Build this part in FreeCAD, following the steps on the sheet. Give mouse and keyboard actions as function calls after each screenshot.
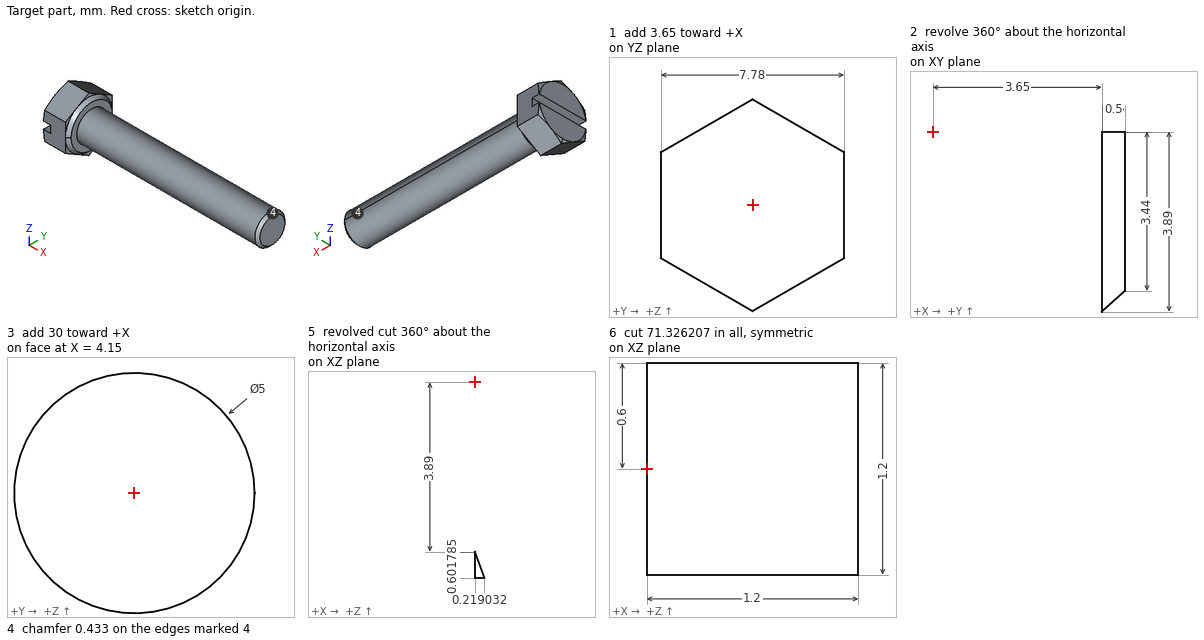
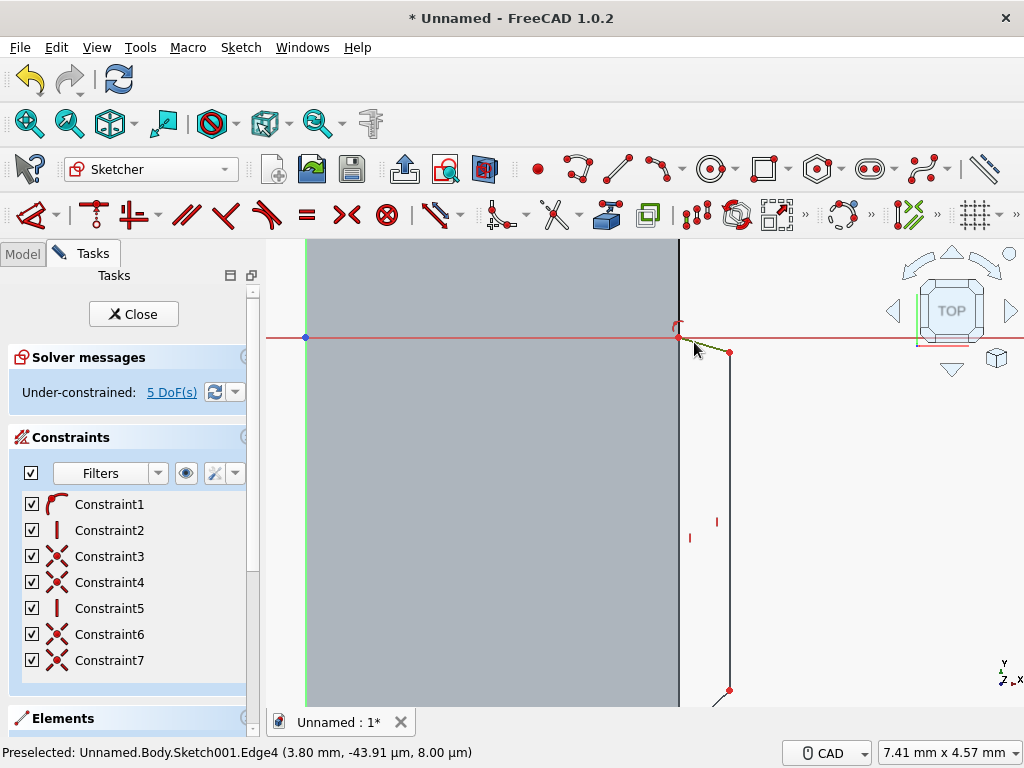
key(h)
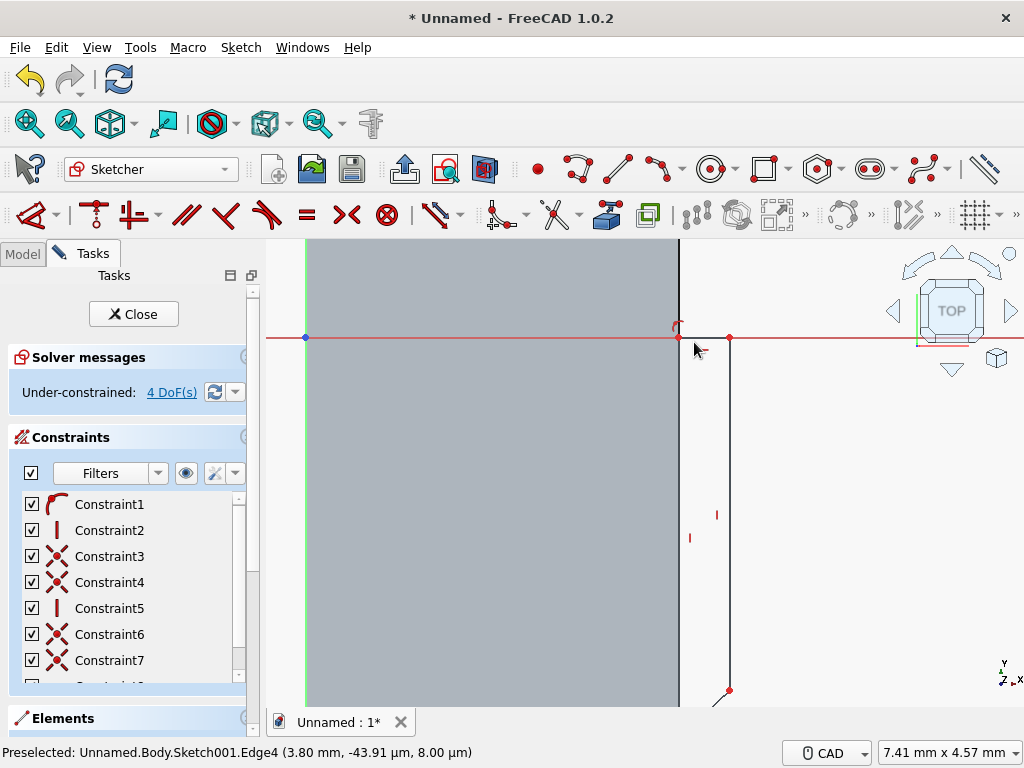
click(714, 338)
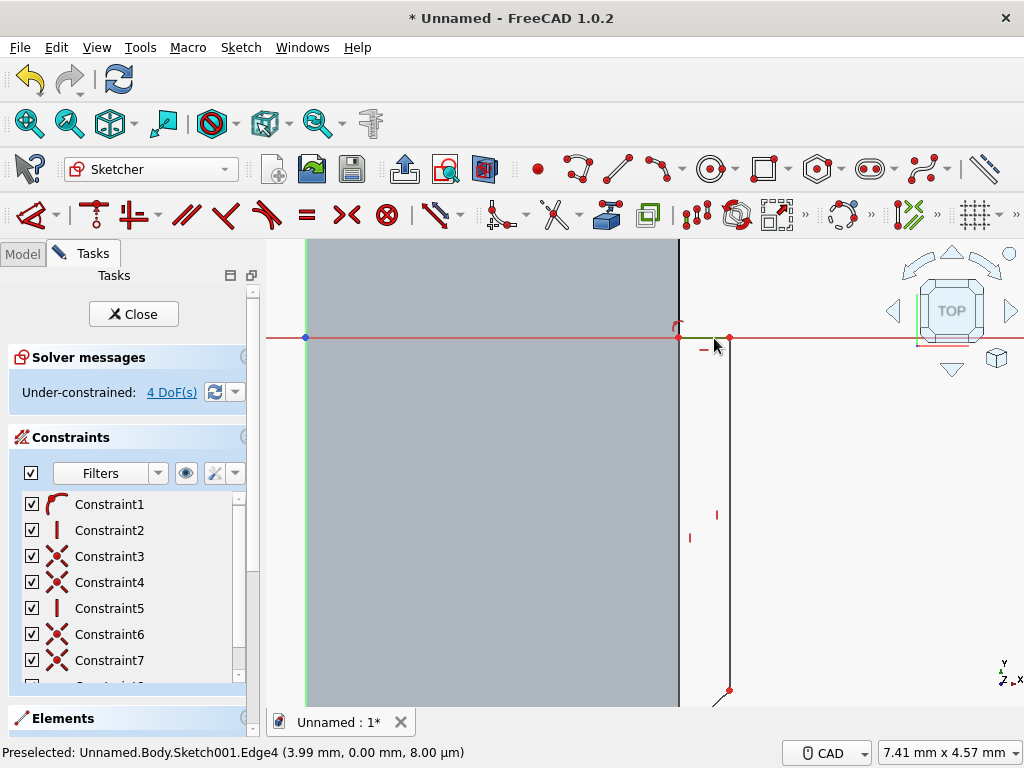
key(l)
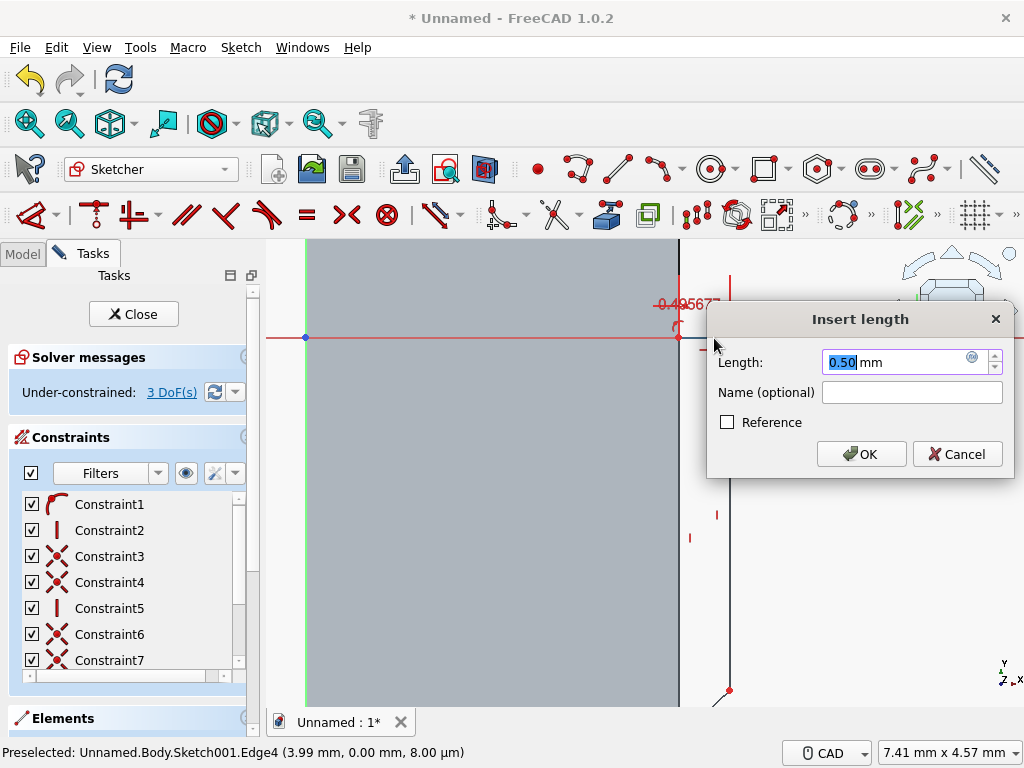
text(0.5)
key(Return)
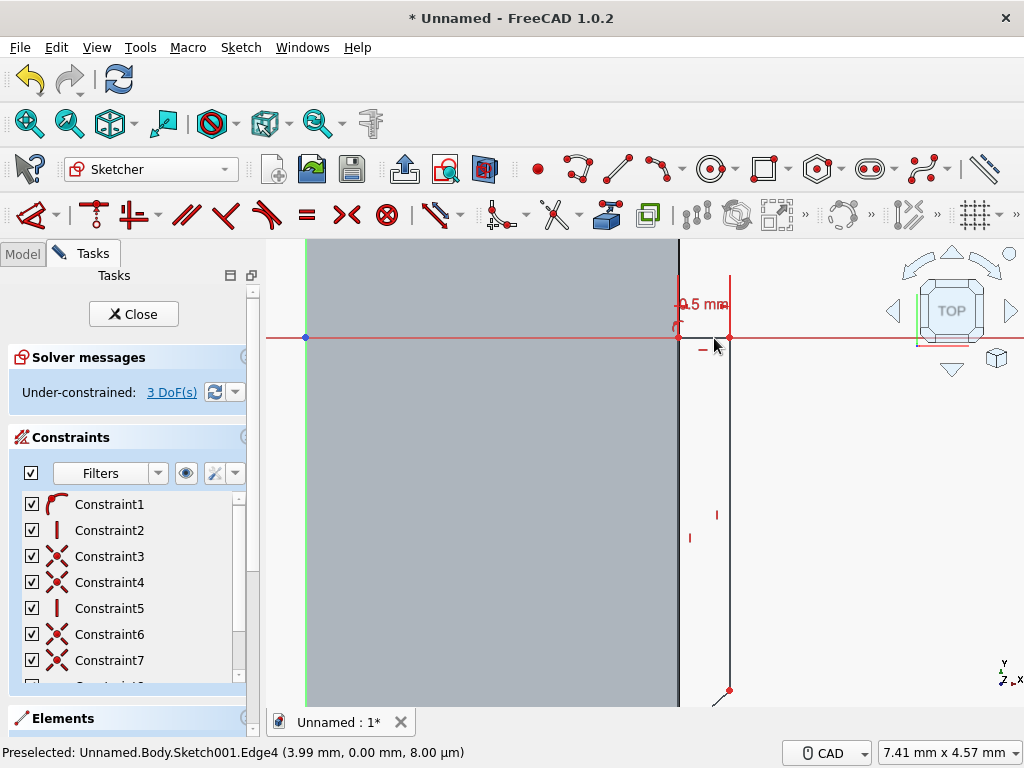
click(678, 457)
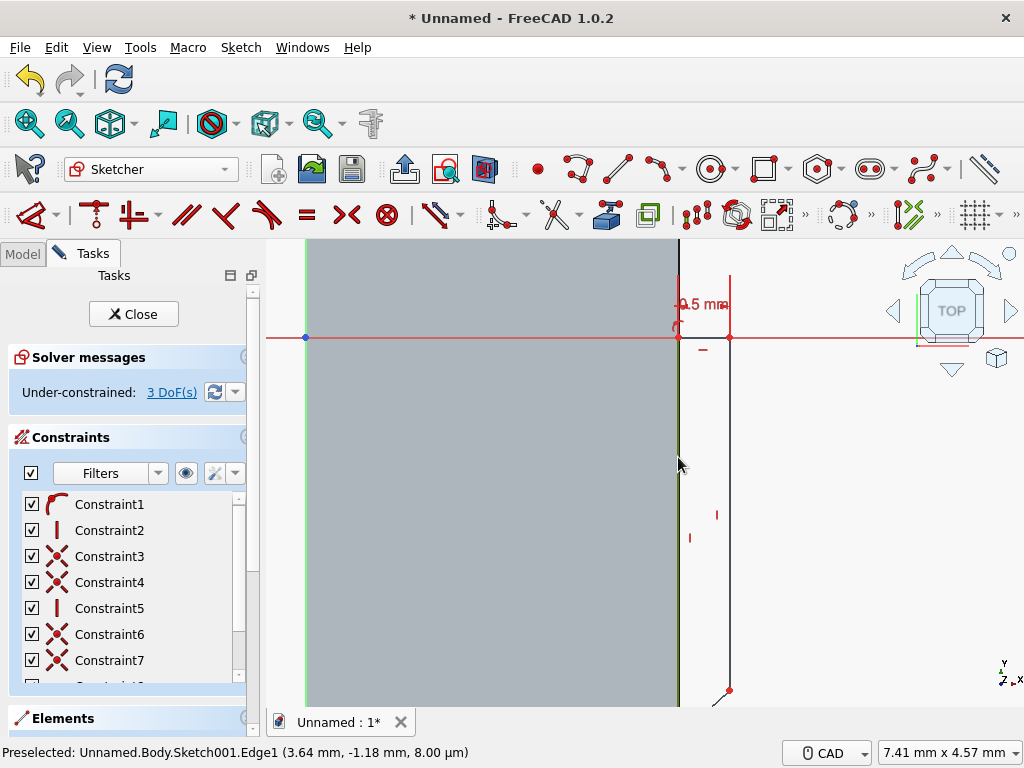
key(i)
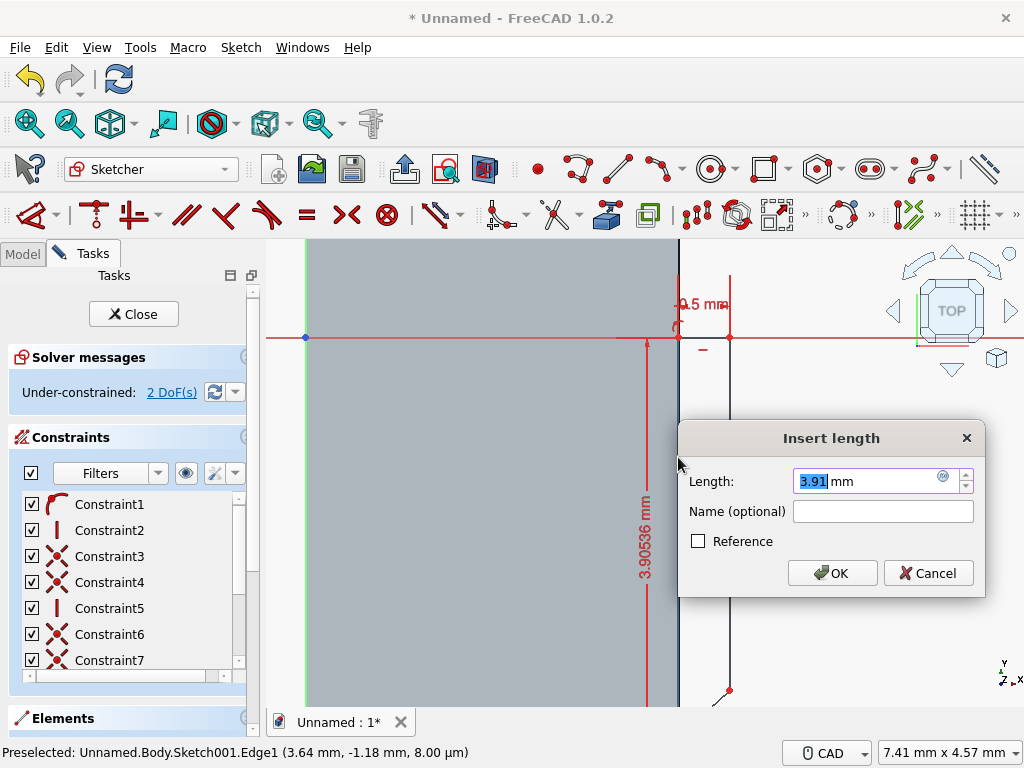
text(3.89)
key(Return)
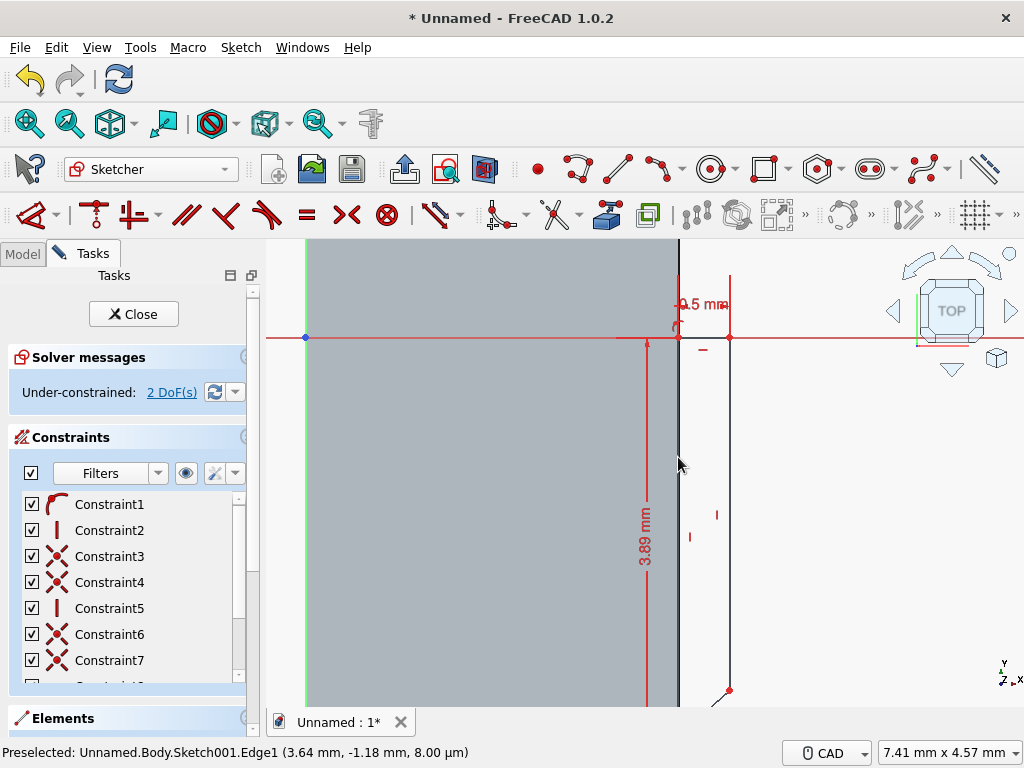
click(730, 585)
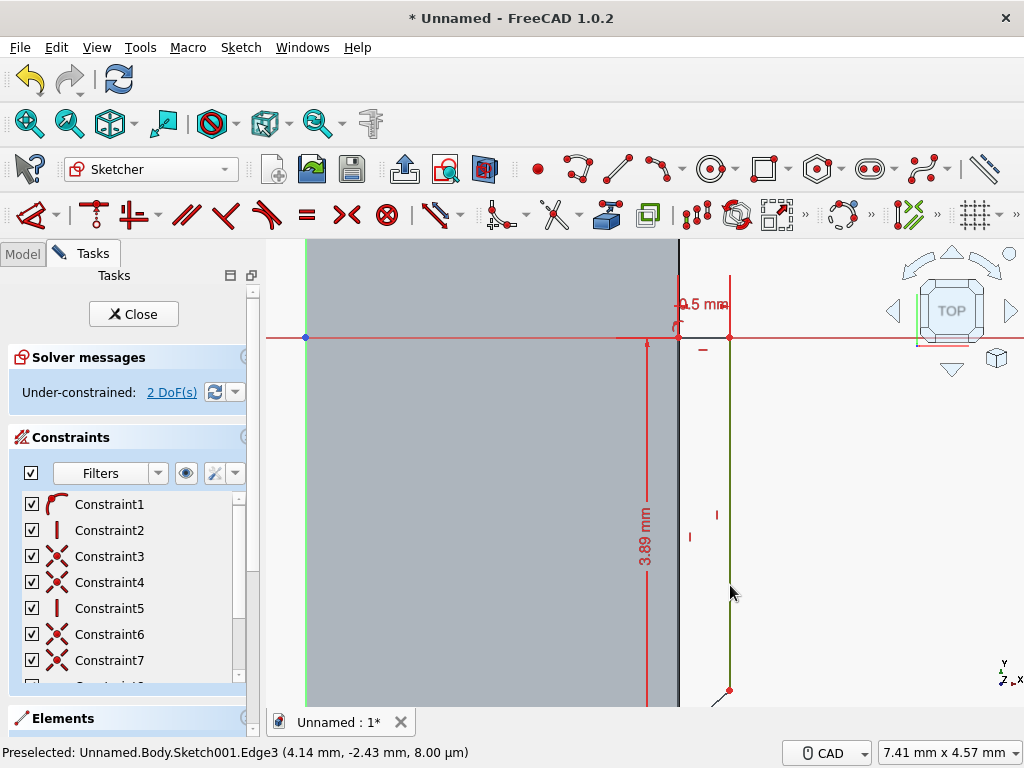
key(i)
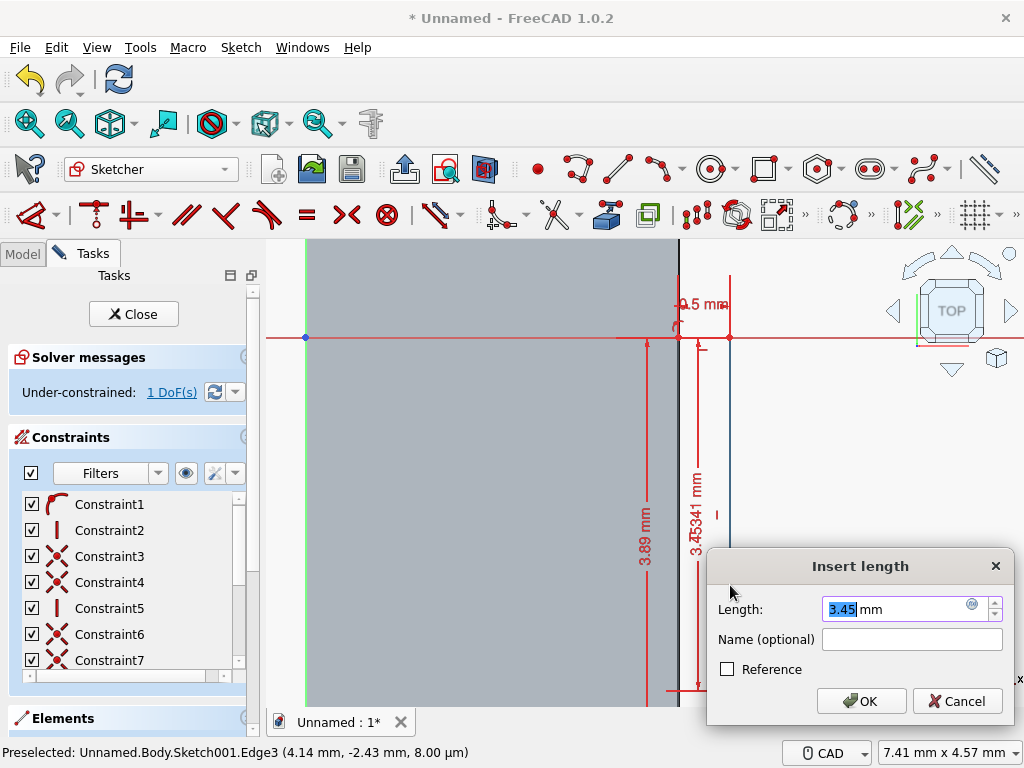
text(3.44)
key(Return)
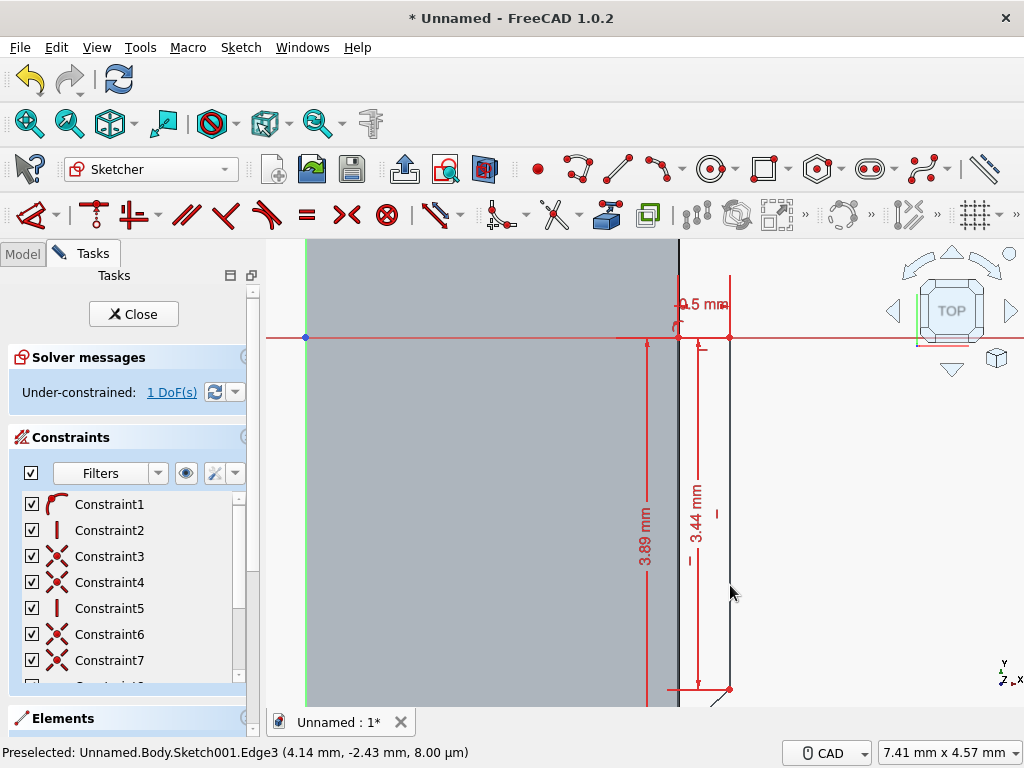
click(678, 338)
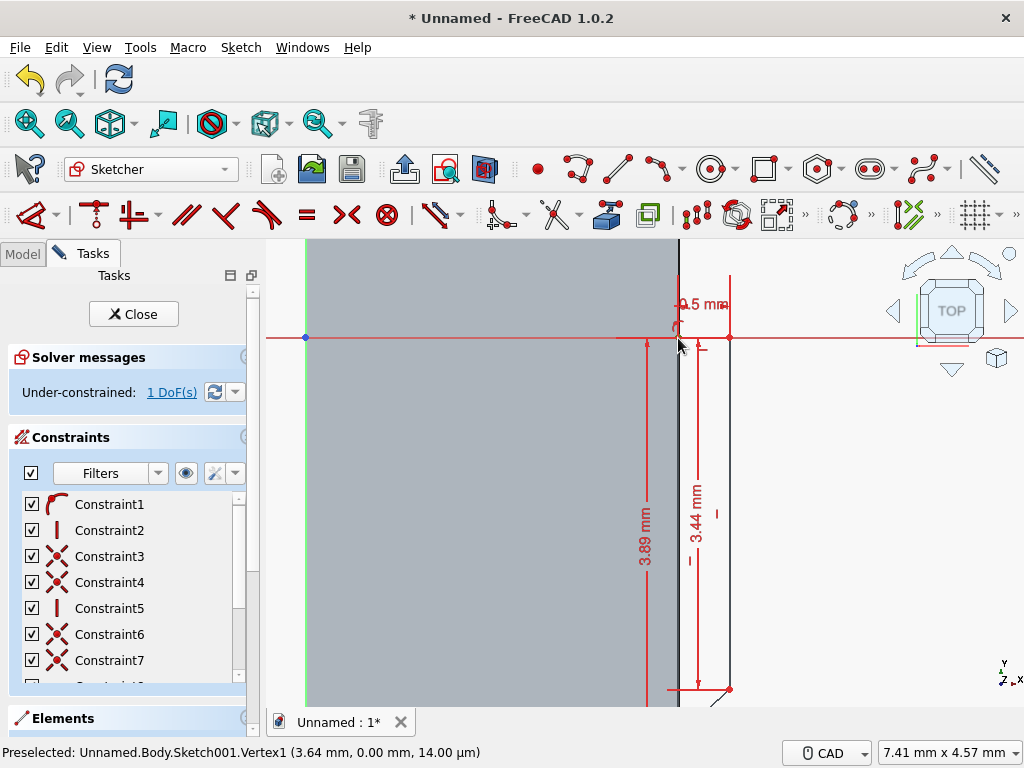
click(58, 216)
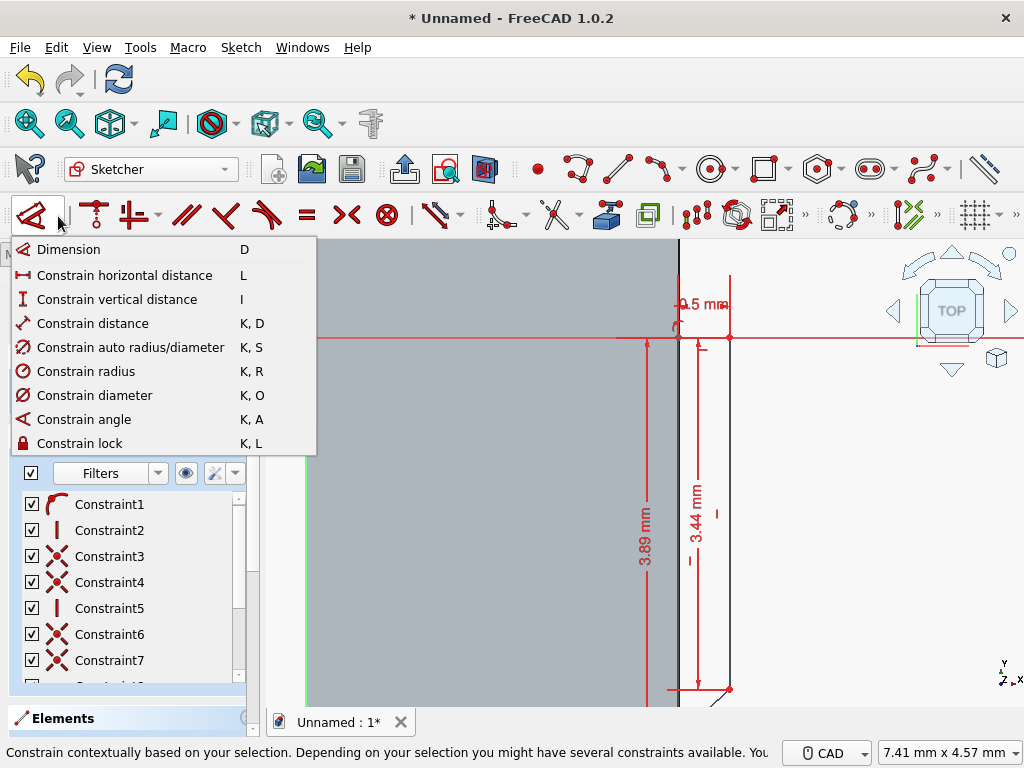
click(164, 275)